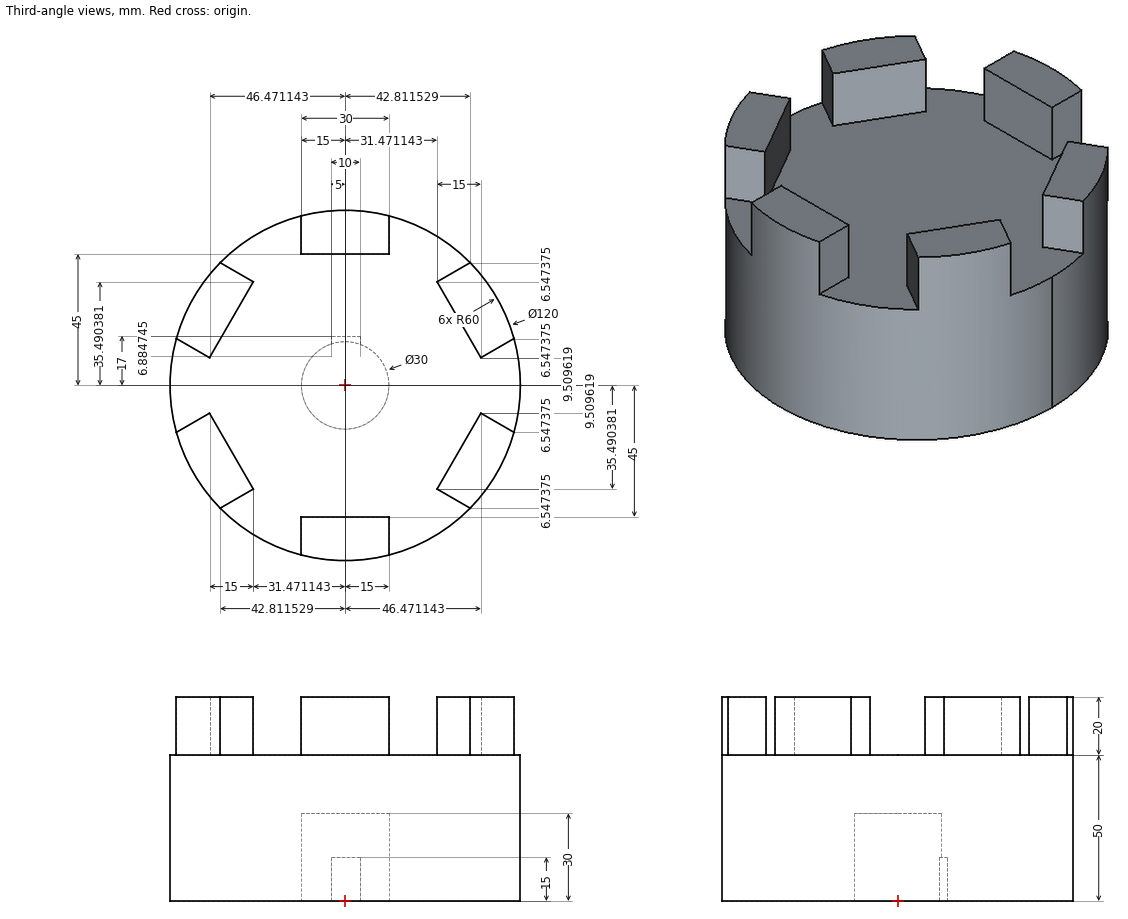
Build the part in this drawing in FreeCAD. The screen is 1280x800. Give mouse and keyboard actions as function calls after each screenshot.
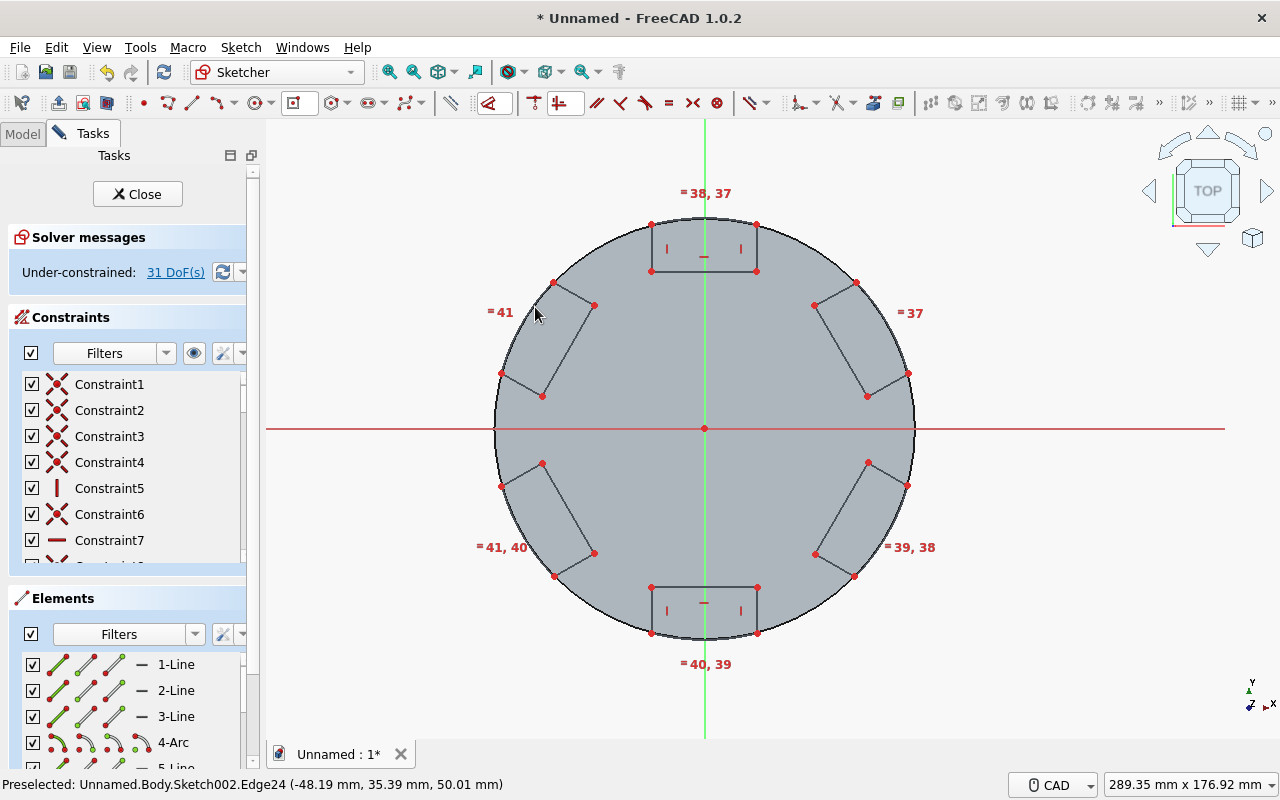
click(898, 344)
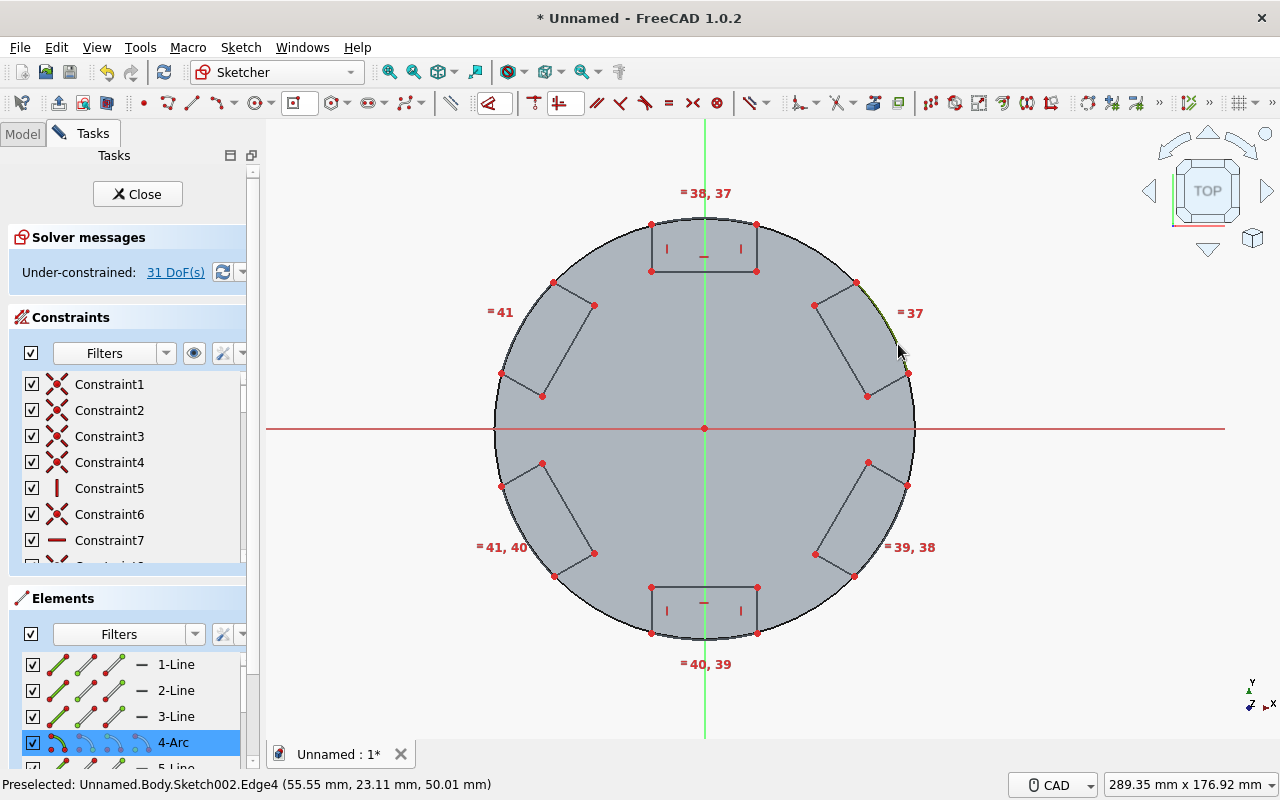
key(k)
key(r)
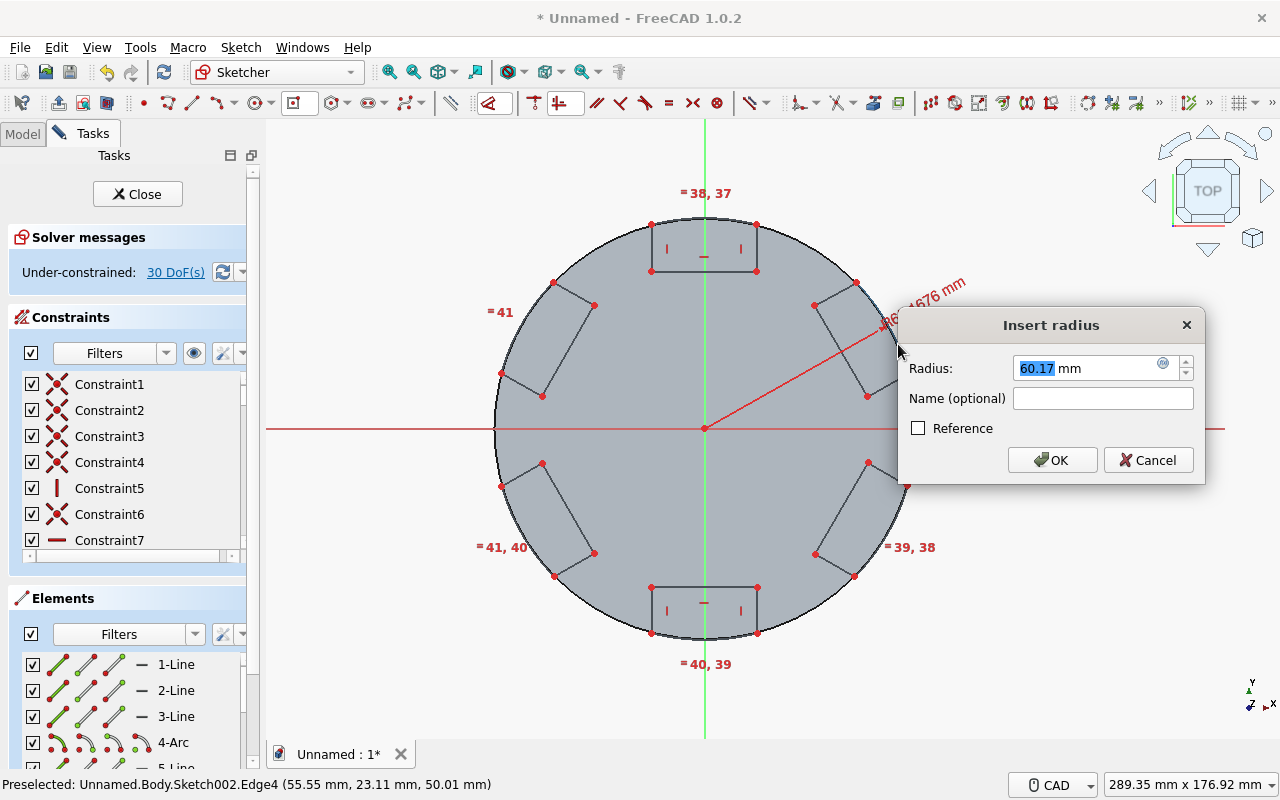
text(60)
key(Return)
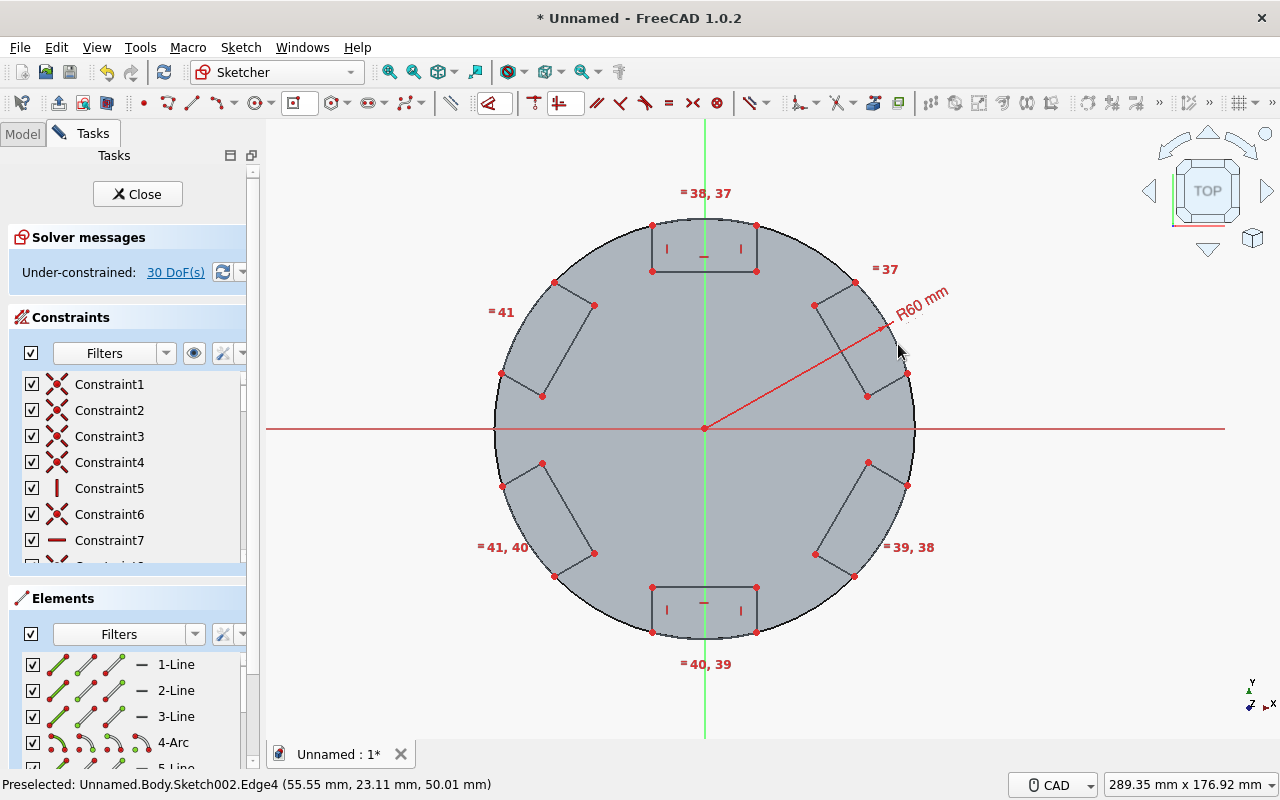
click(684, 272)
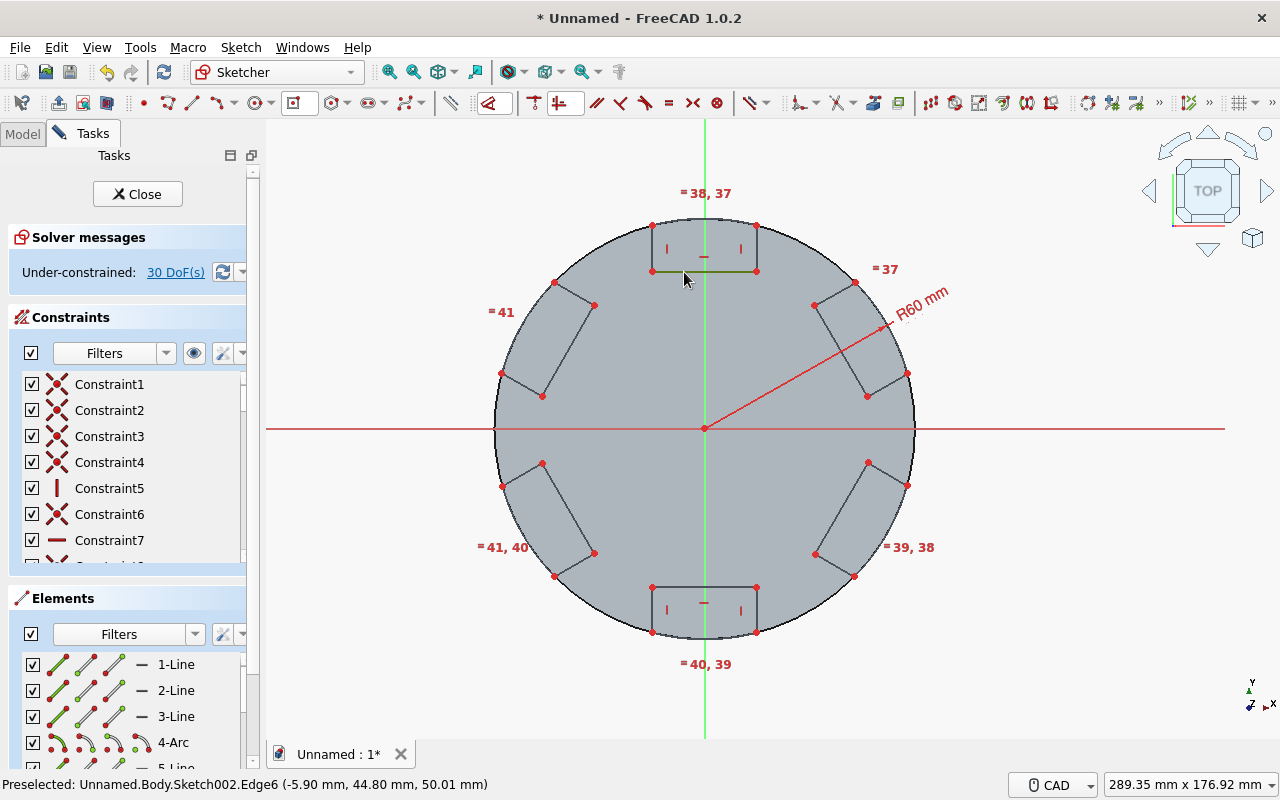
key(l)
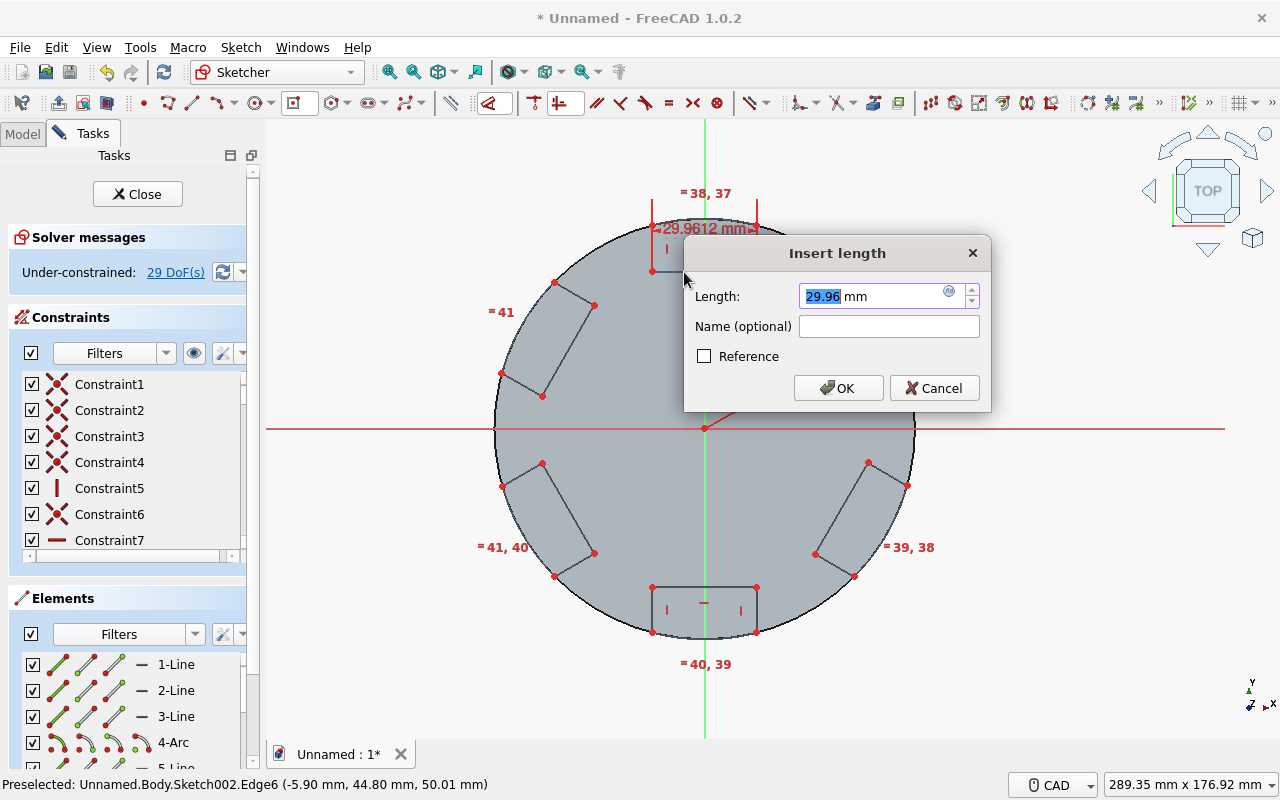
text(30)
key(Return)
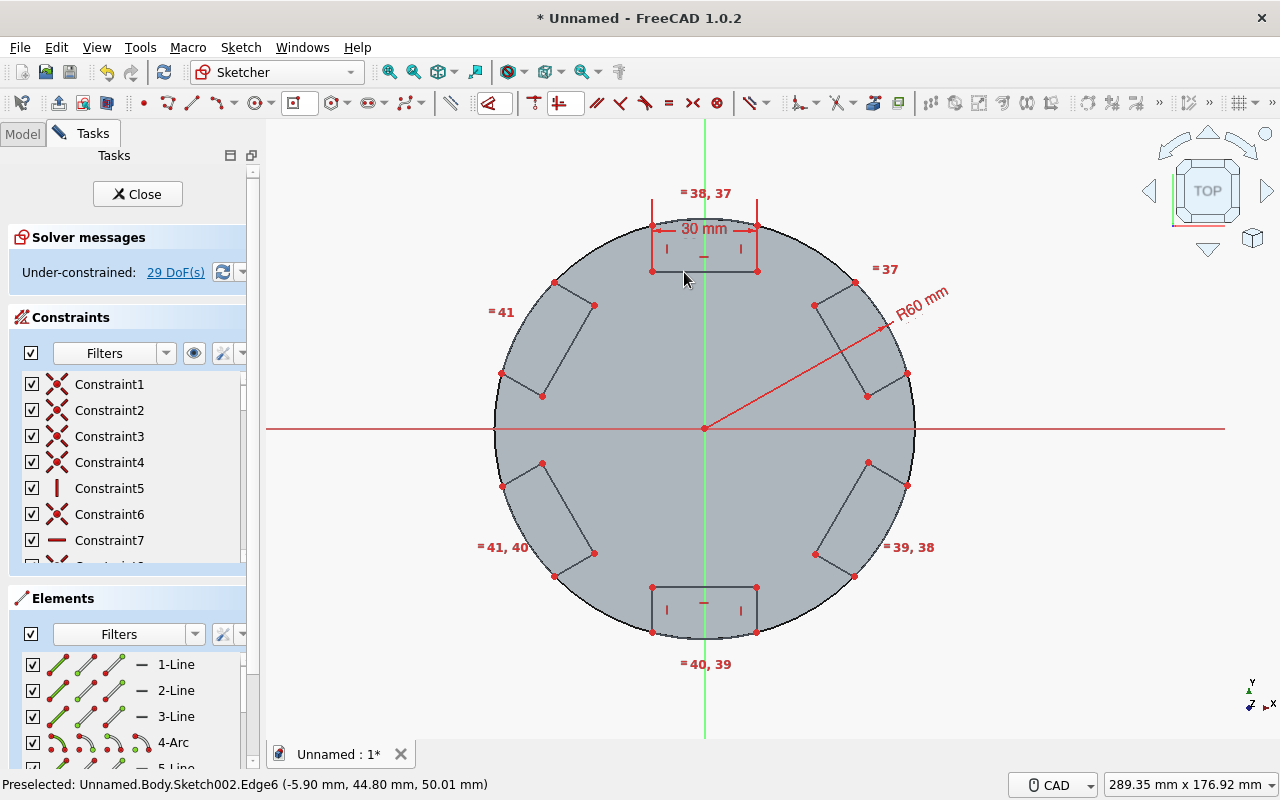
click(726, 587)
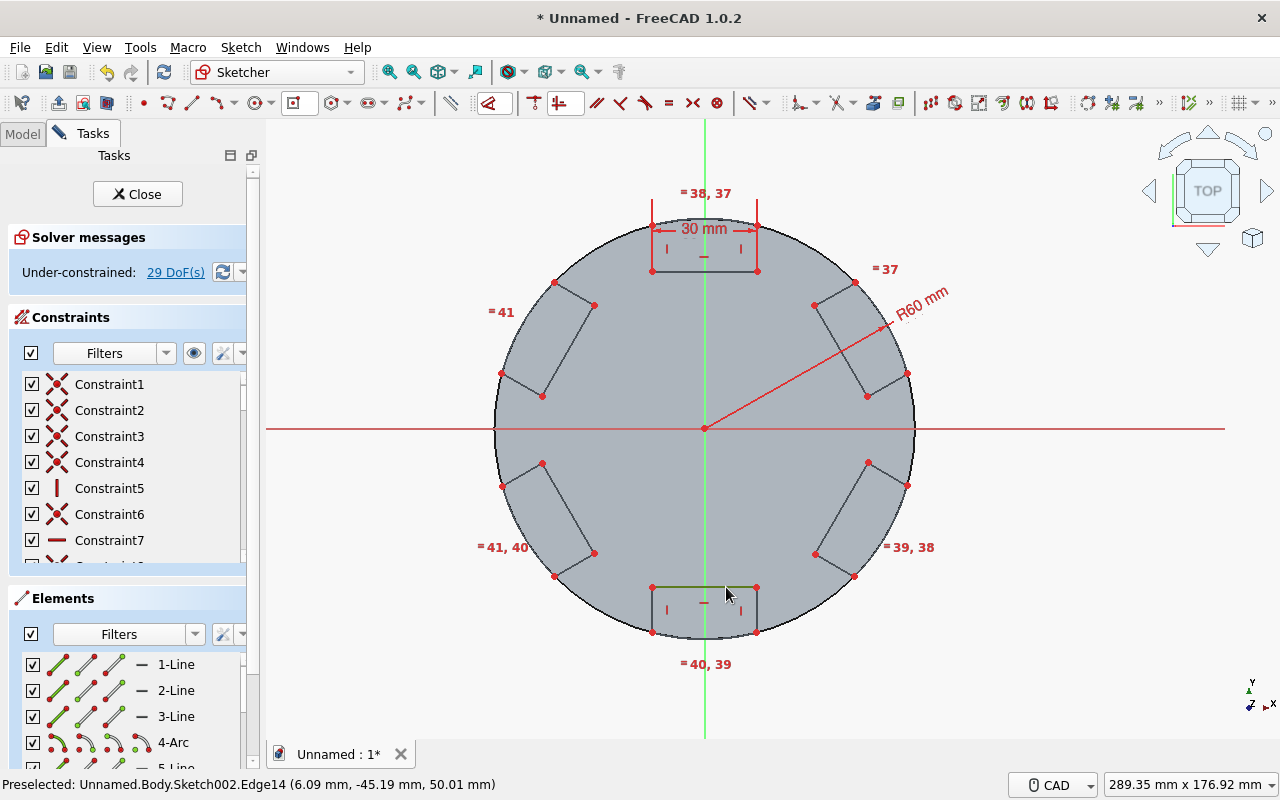
key(l)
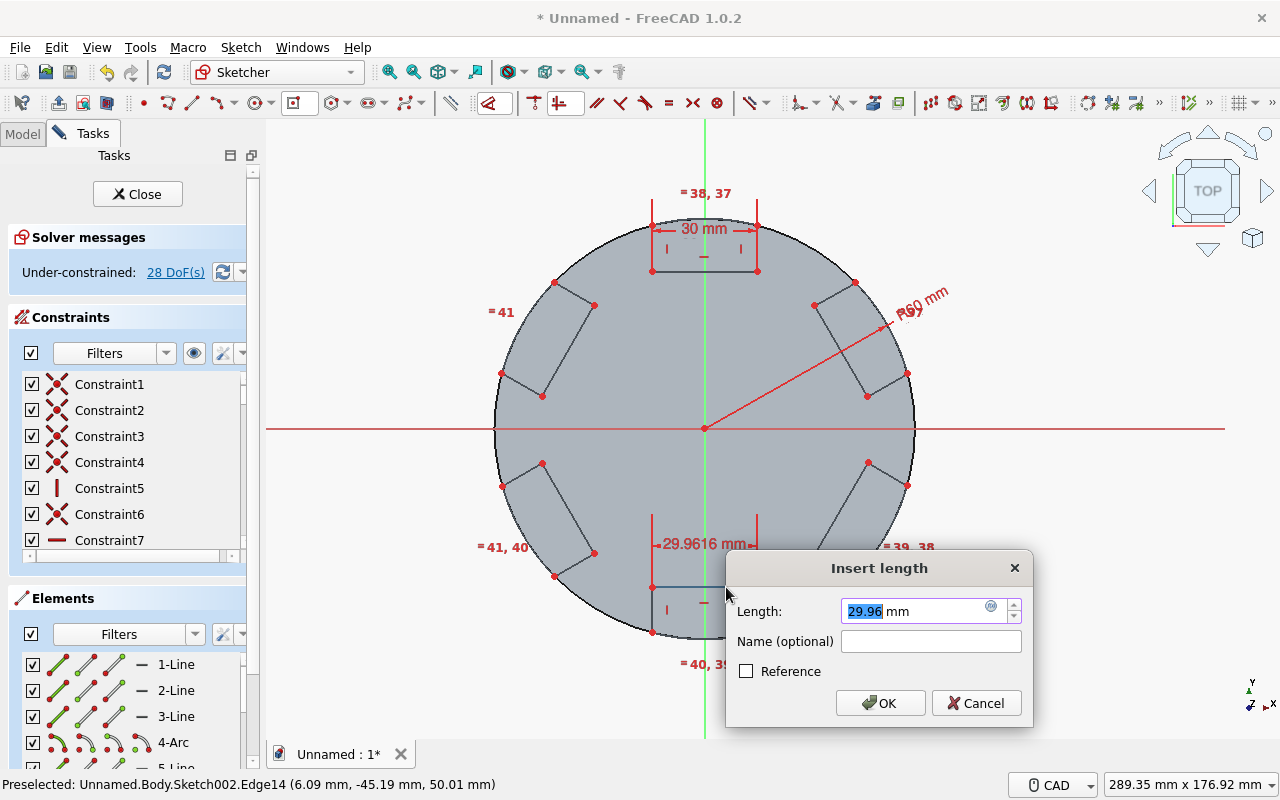
text(30)
key(Return)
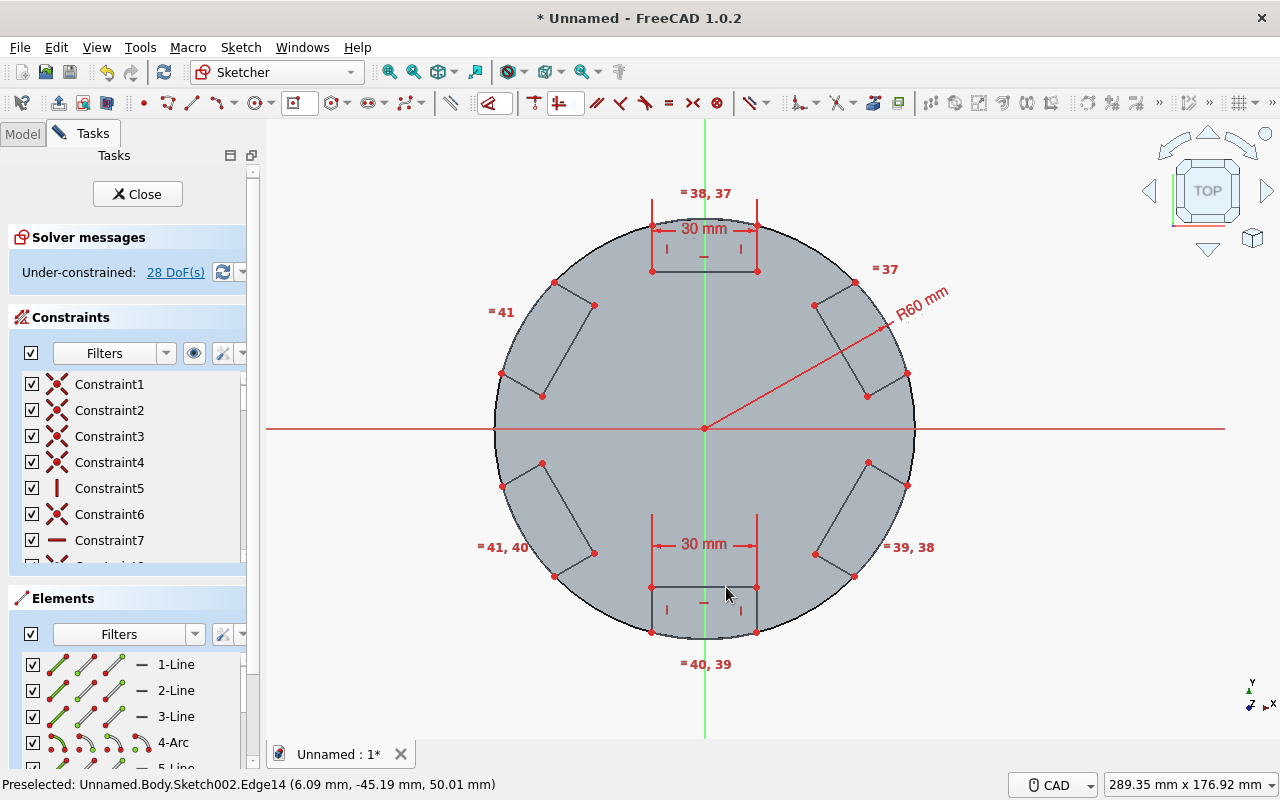
click(652, 225)